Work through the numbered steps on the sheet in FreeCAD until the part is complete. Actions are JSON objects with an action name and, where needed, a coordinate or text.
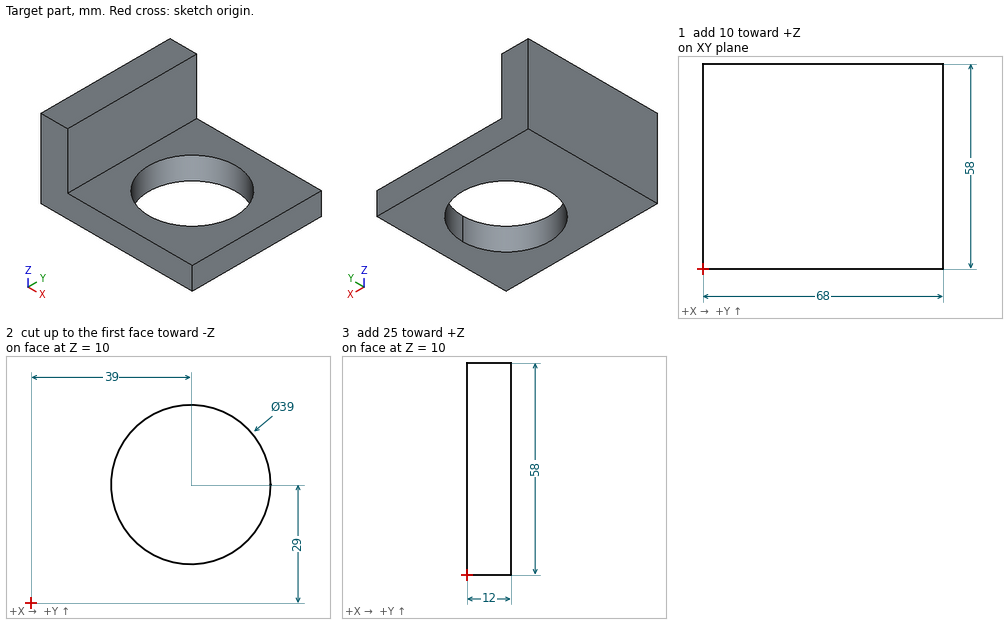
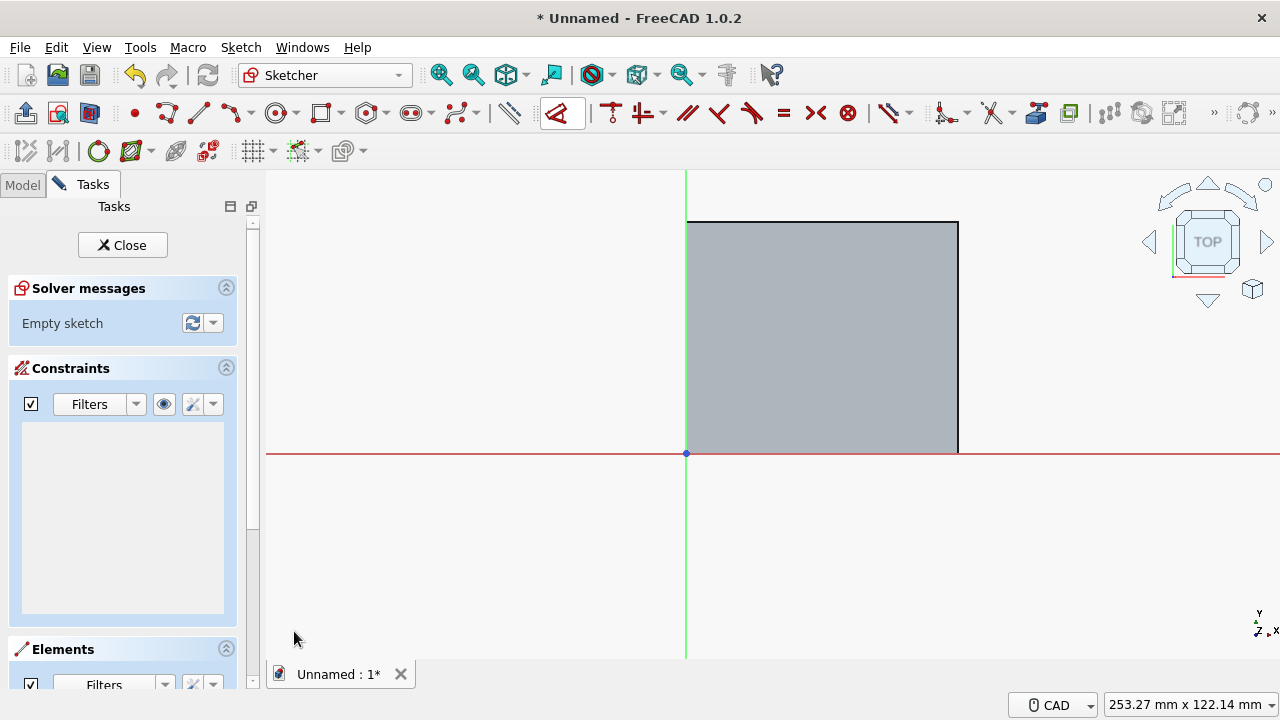
{"action": "scroll", "coordinate": [1004, 240], "scroll_direction": "up", "scroll_amount": 2}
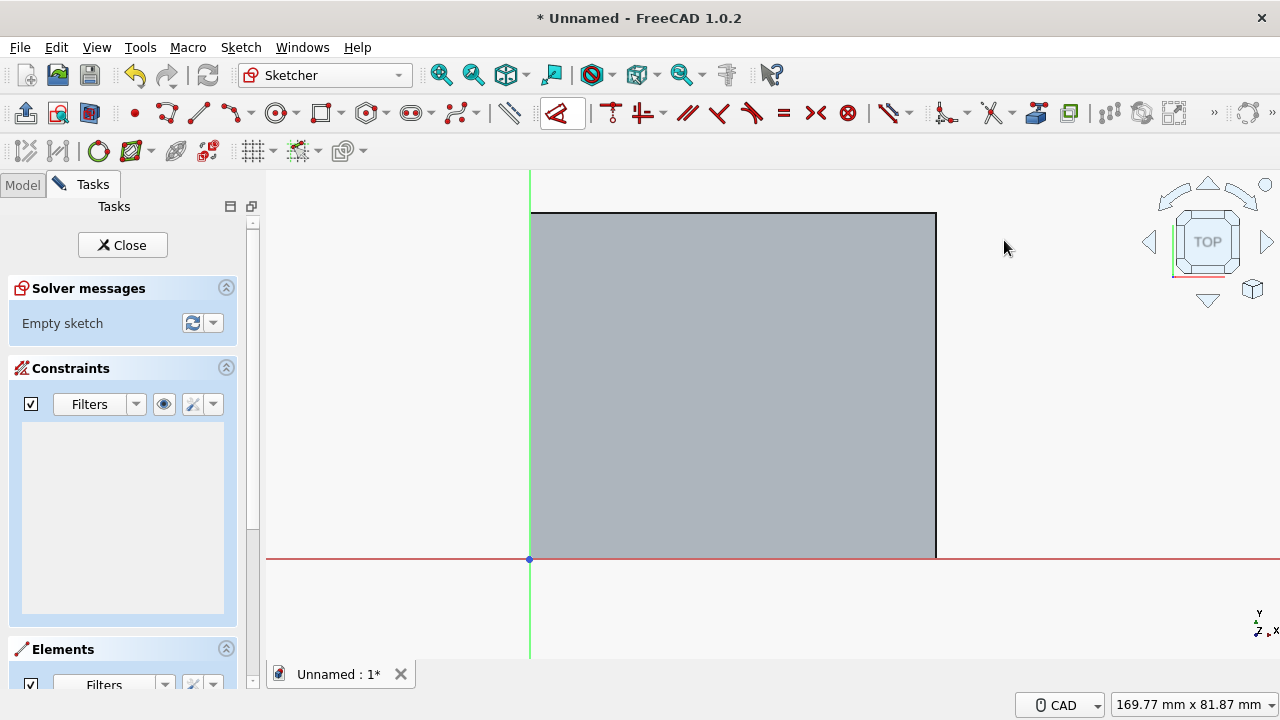
{"action": "key", "text": "g c"}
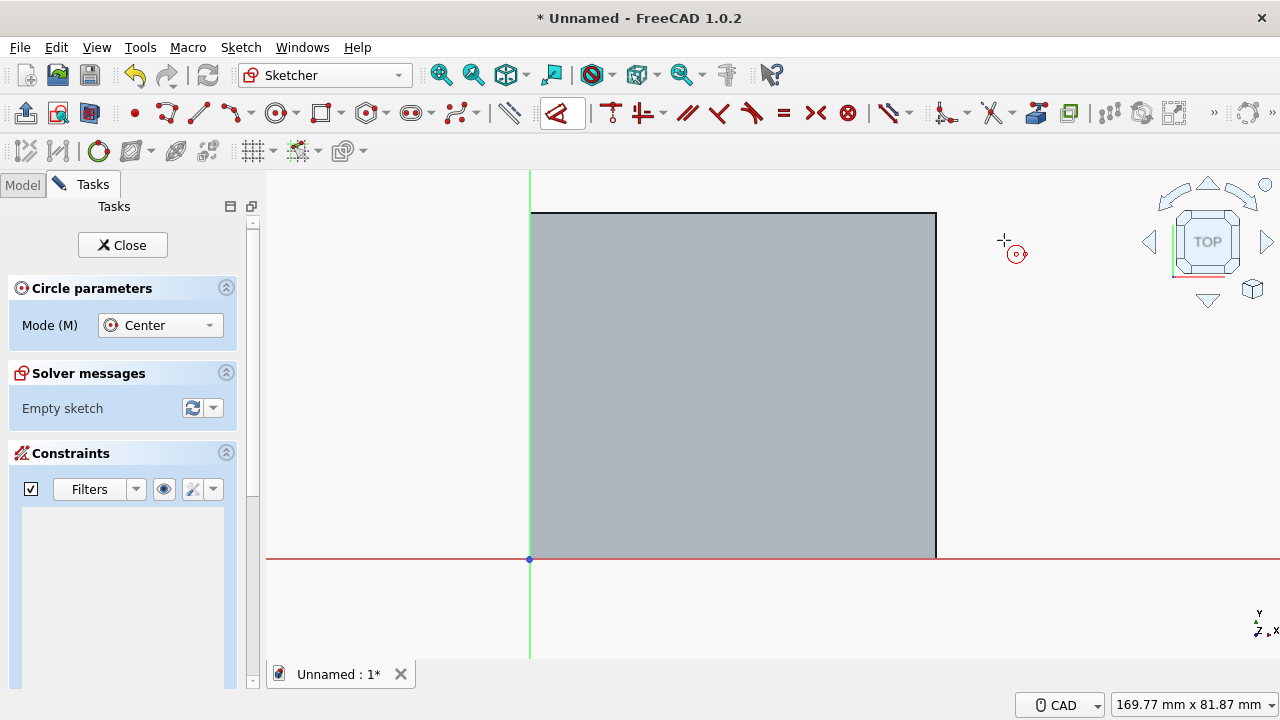
{"action": "left_click", "coordinate": [762, 386]}
{"action": "left_click", "coordinate": [845, 303]}
{"action": "key", "text": "Escape"}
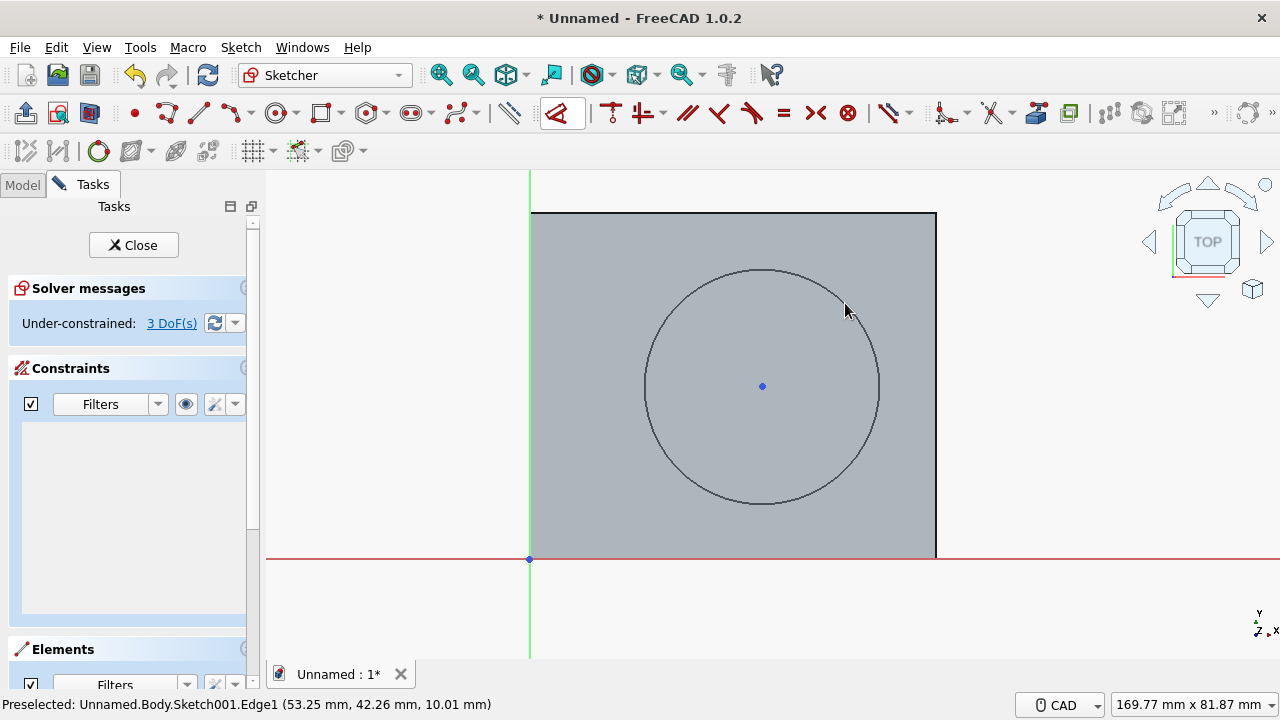
{"action": "left_click", "coordinate": [845, 304]}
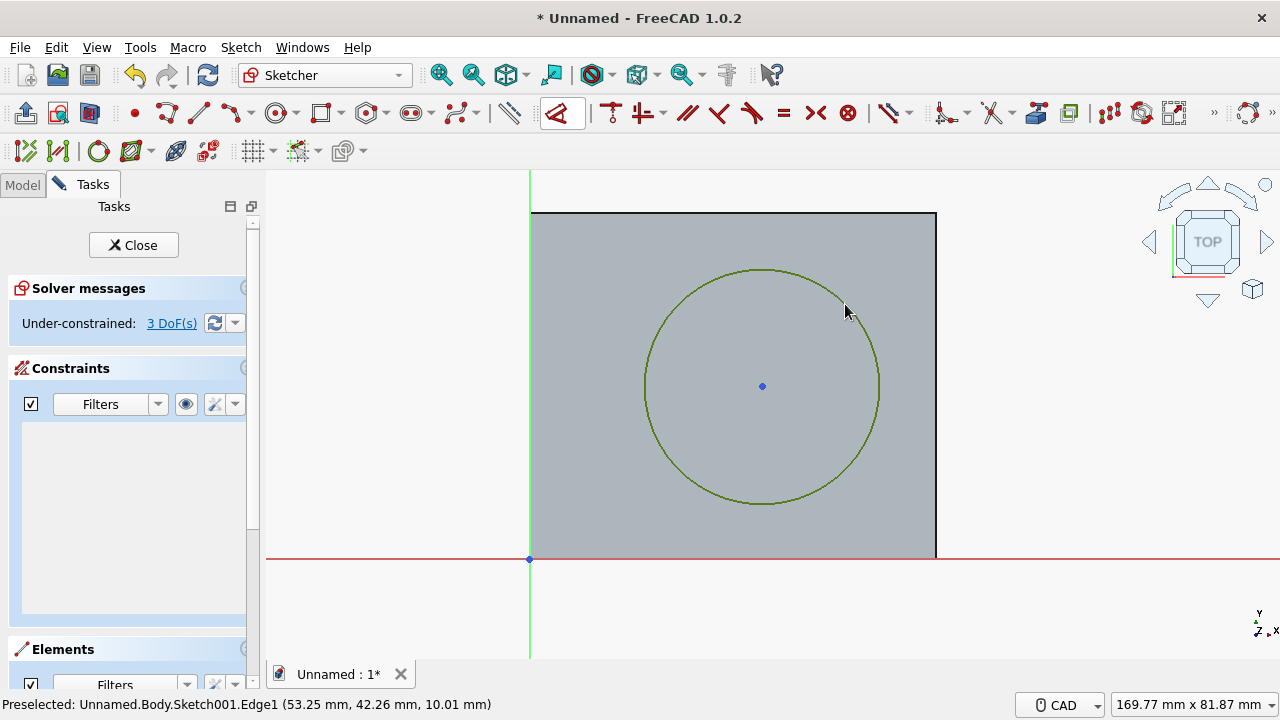
{"action": "key", "text": "k o"}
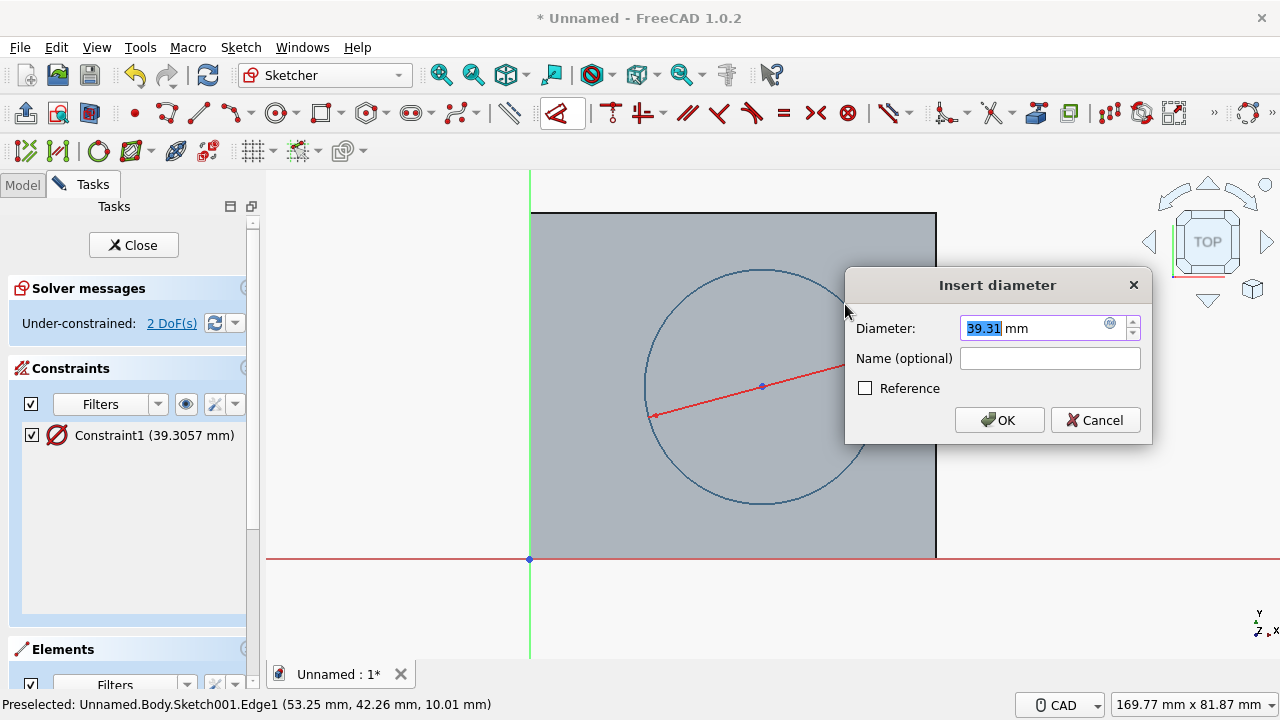
{"action": "type", "text": "39"}
{"action": "key", "text": "Return"}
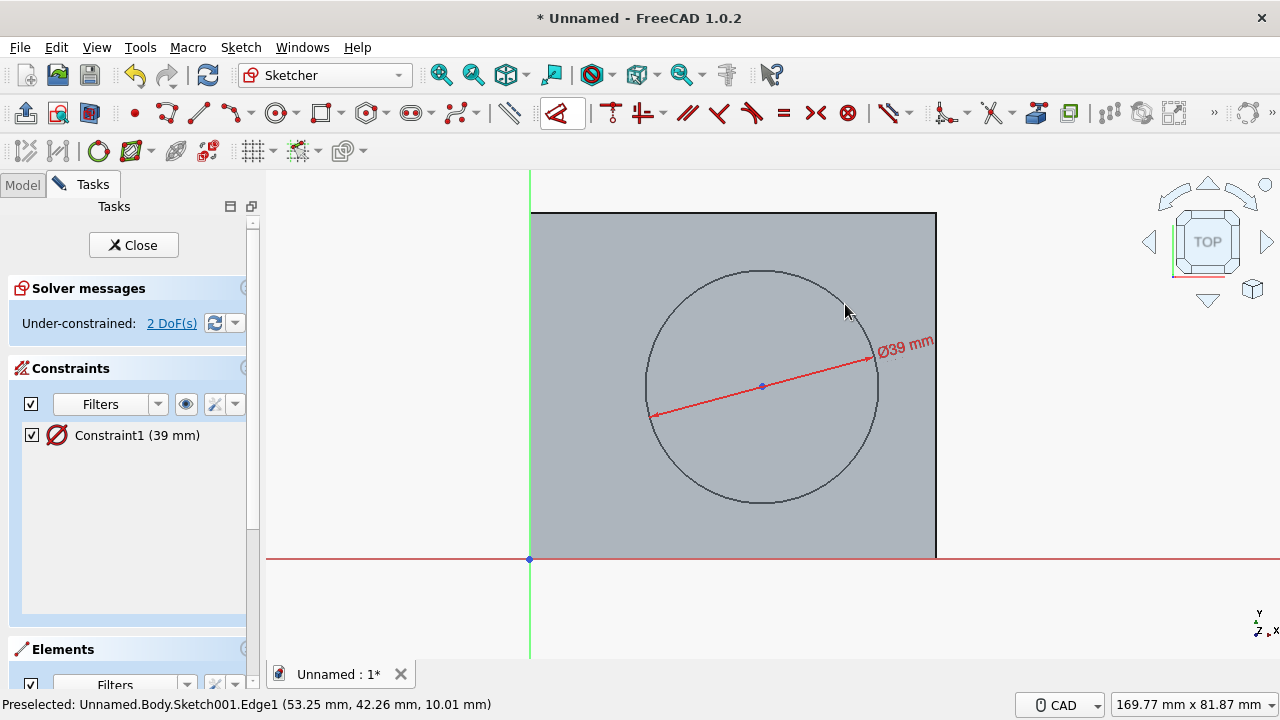
{"action": "left_click", "coordinate": [762, 387]}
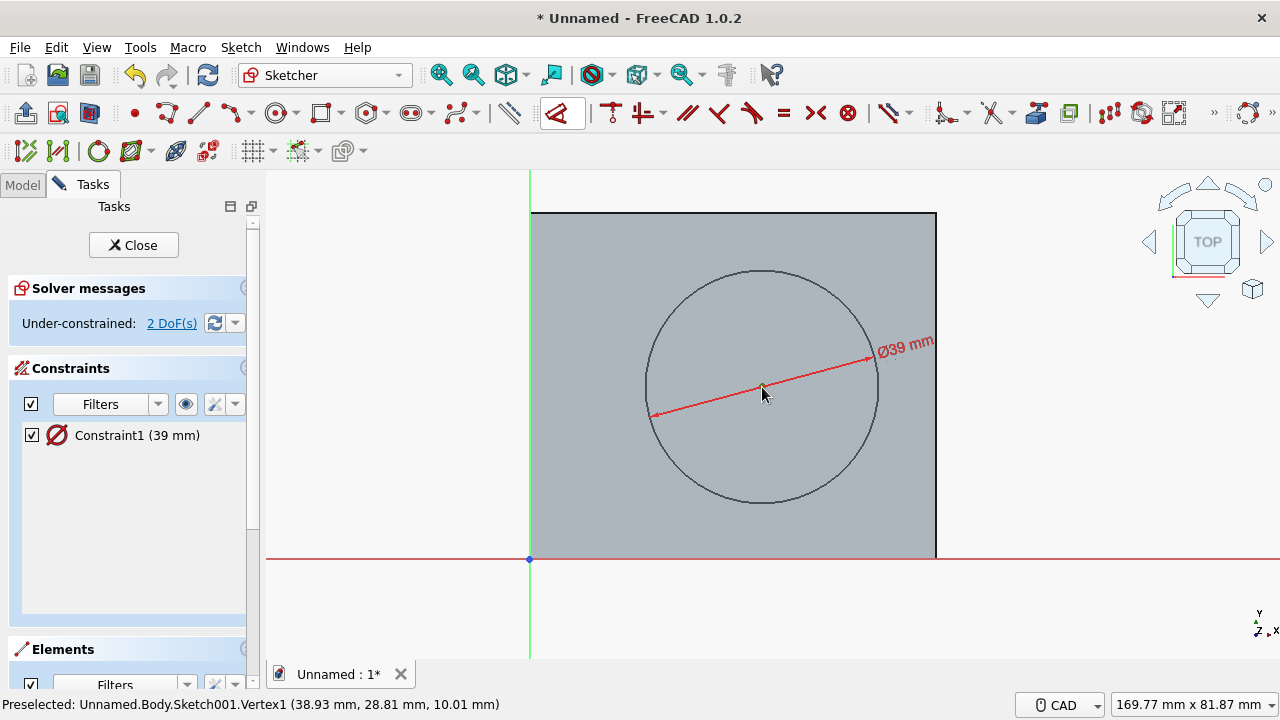
{"action": "left_click", "coordinate": [580, 114]}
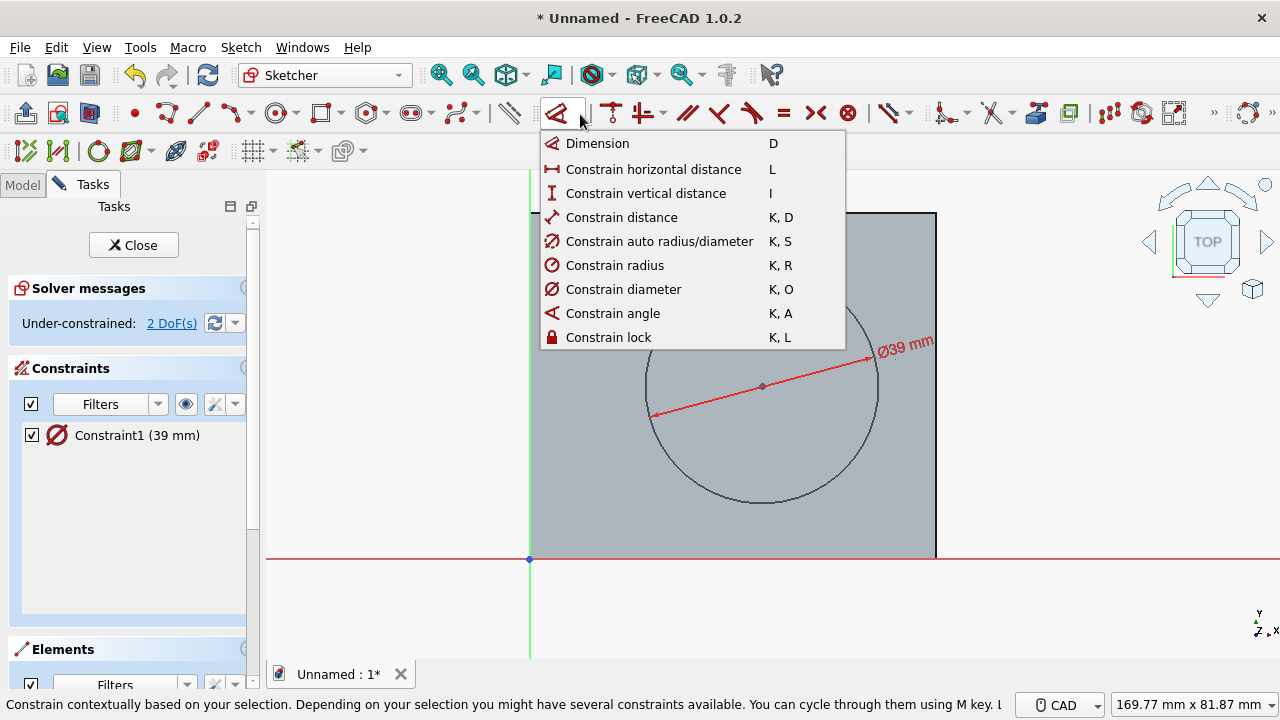
{"action": "left_click", "coordinate": [693, 169]}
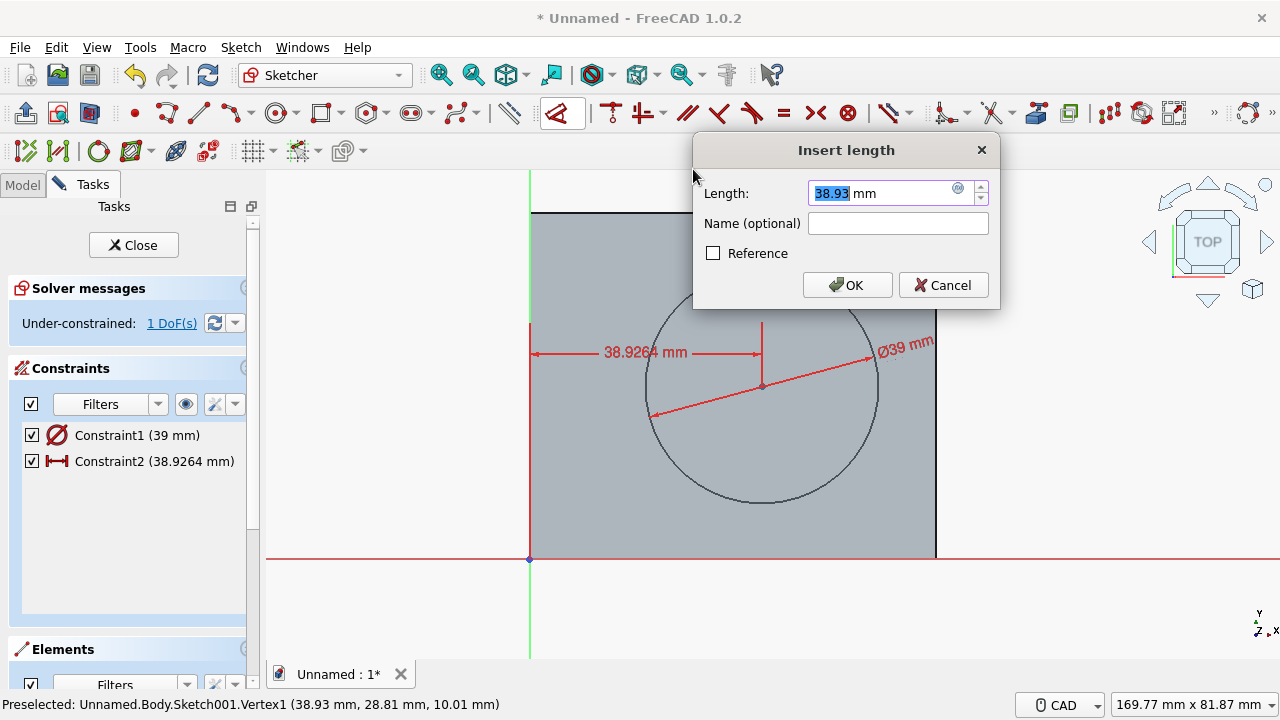
{"action": "type", "text": "39"}
{"action": "key", "text": "Return"}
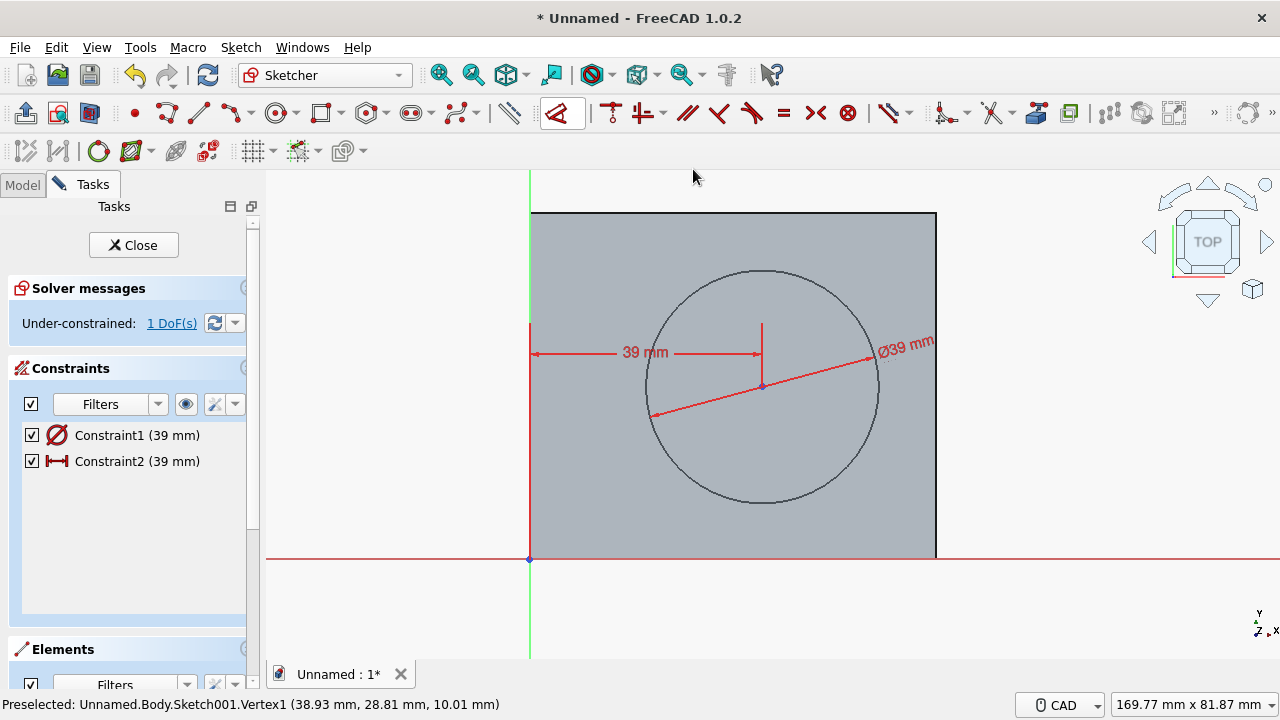
{"action": "left_click", "coordinate": [762, 387]}